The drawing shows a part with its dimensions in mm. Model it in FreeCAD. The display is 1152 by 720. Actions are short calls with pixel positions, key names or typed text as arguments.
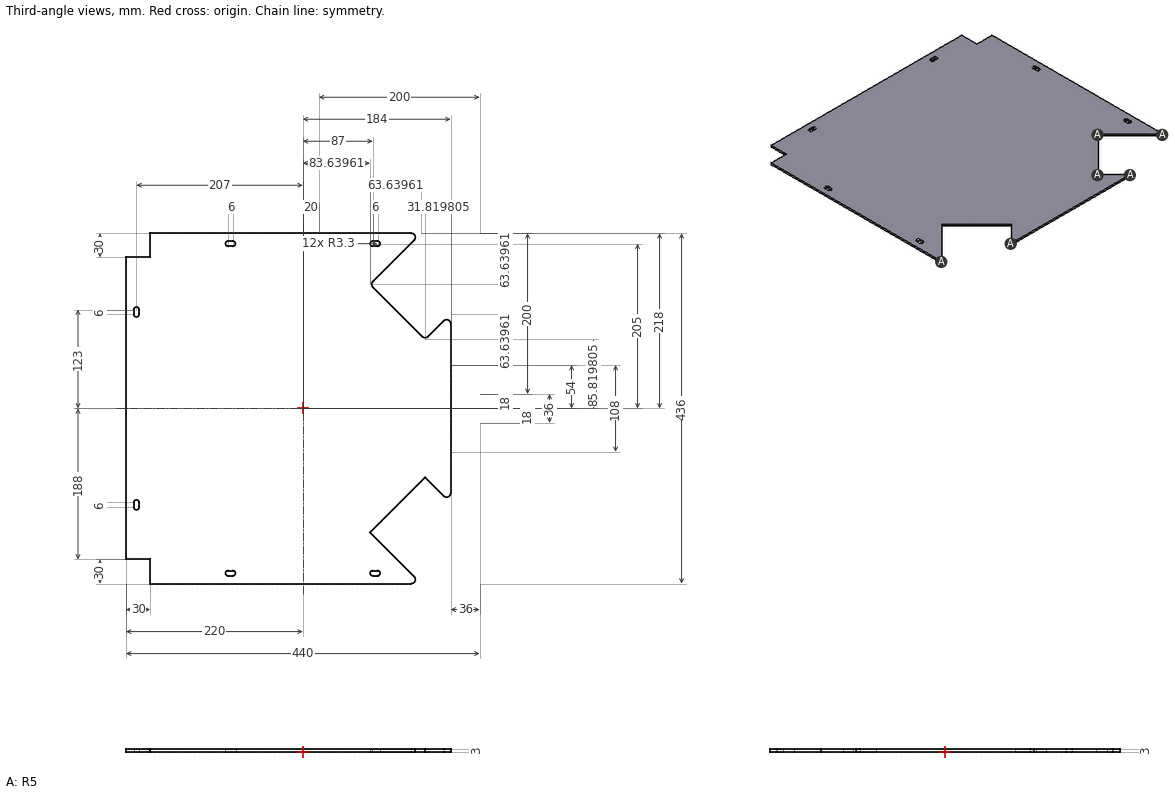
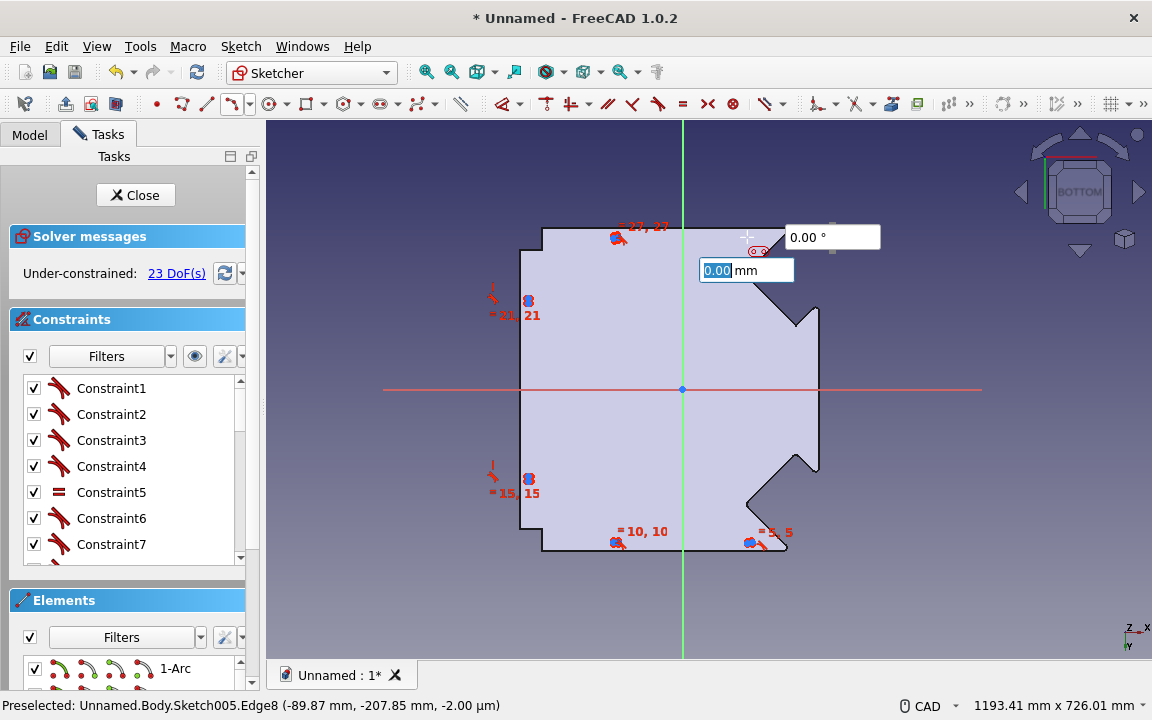
scroll(752, 237, up, 7)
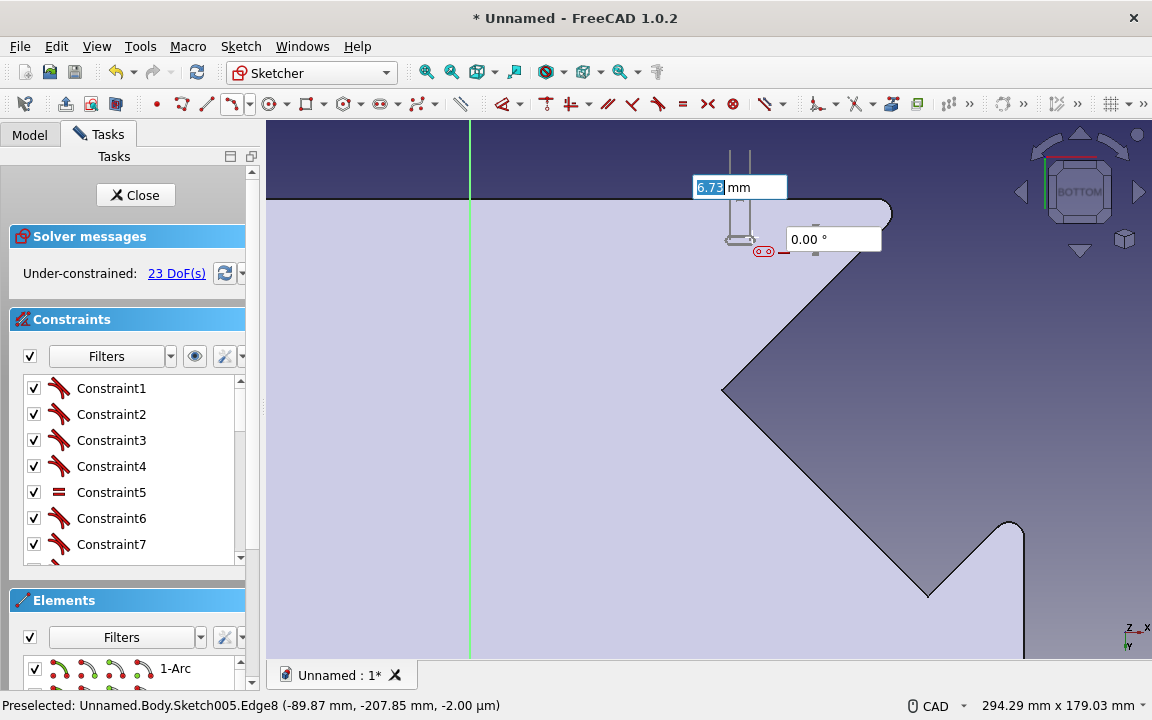
click(750, 236)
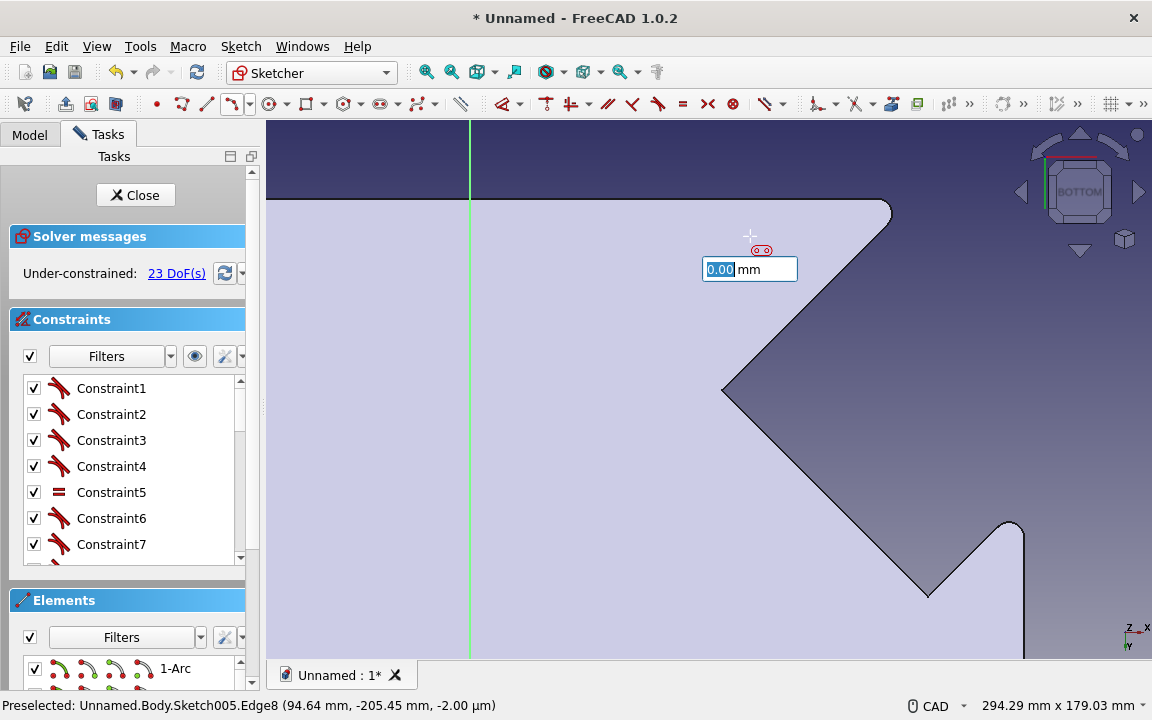
scroll(741, 248, up, 3)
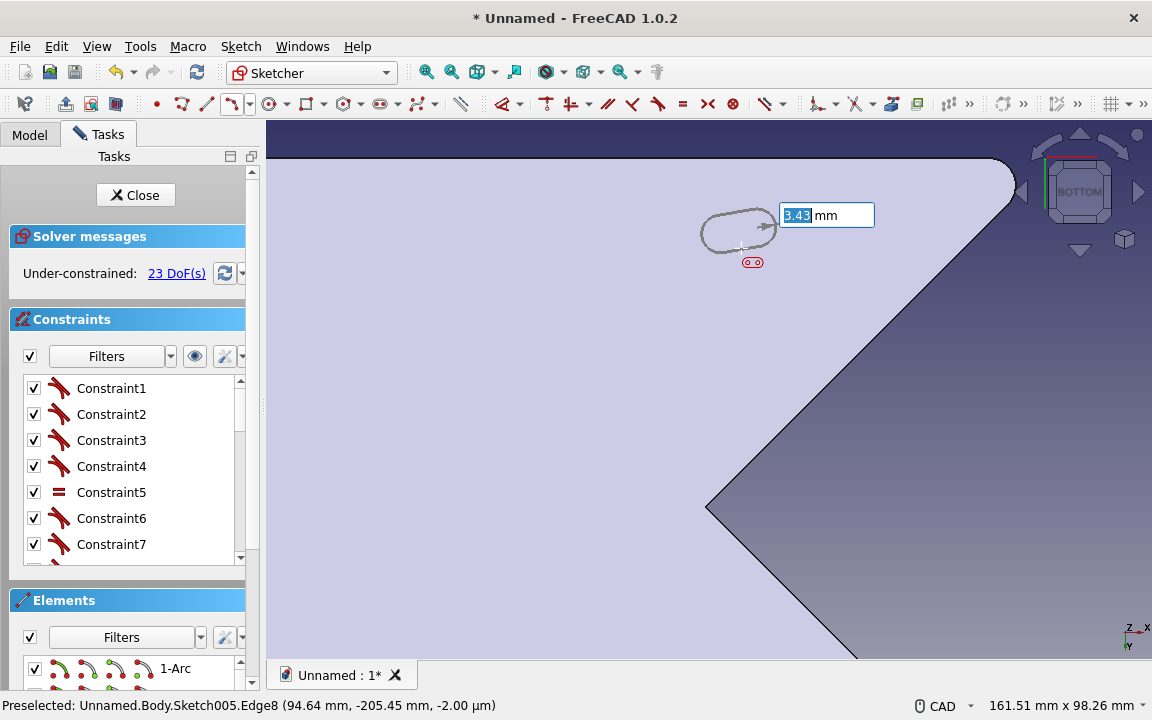
click(740, 247)
key(Escape)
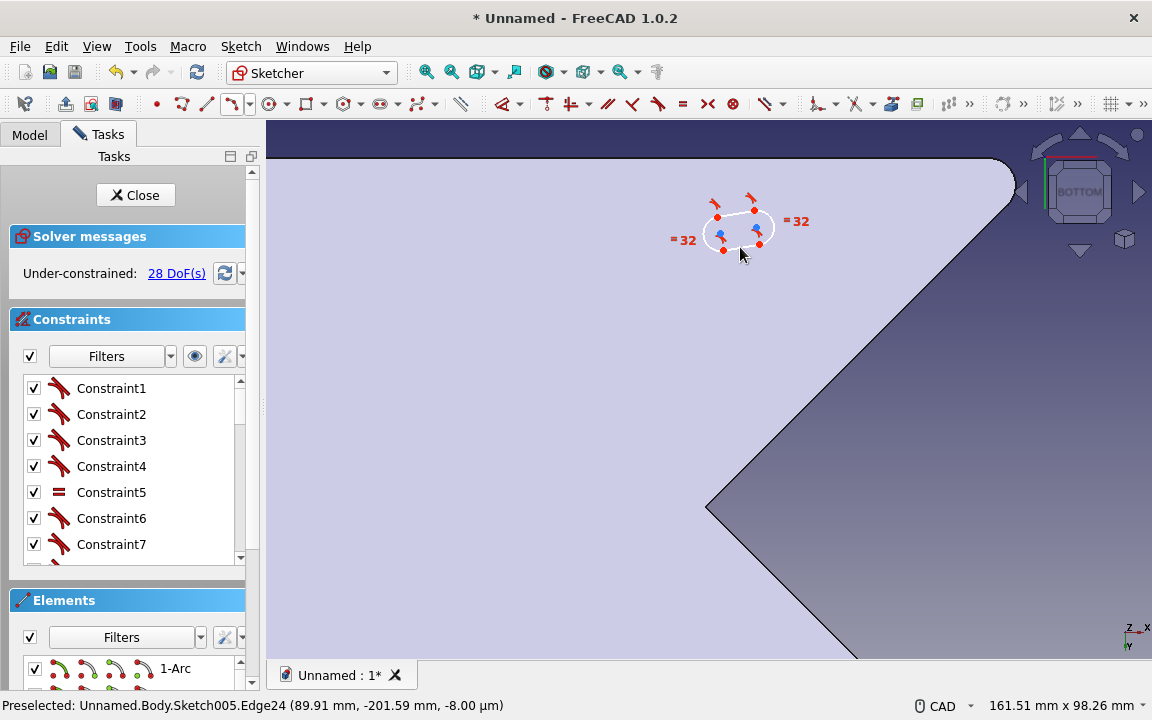
scroll(751, 239, down, 10)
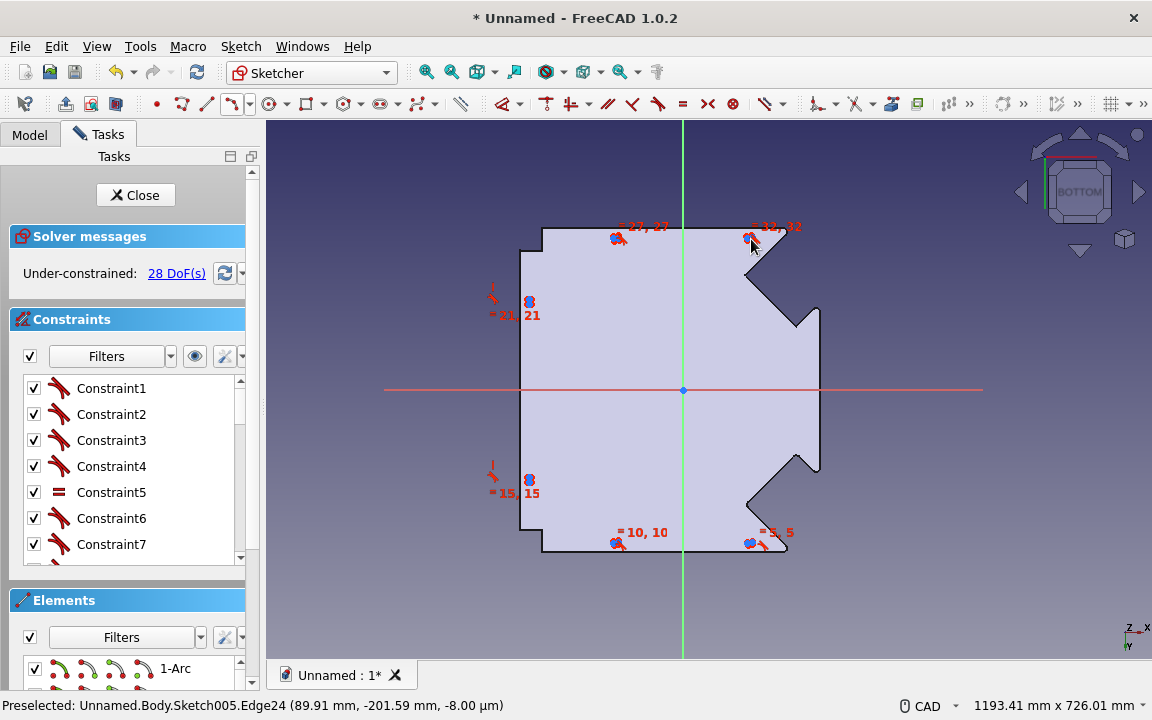
scroll(749, 542, up, 12)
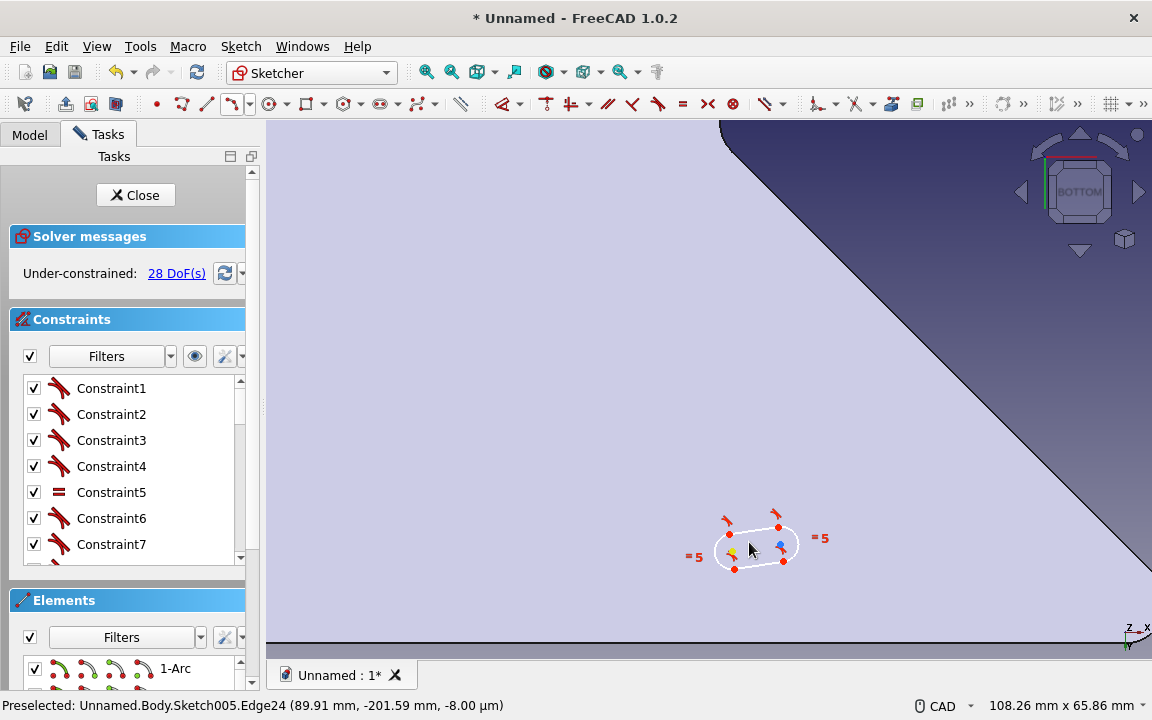
click(744, 532)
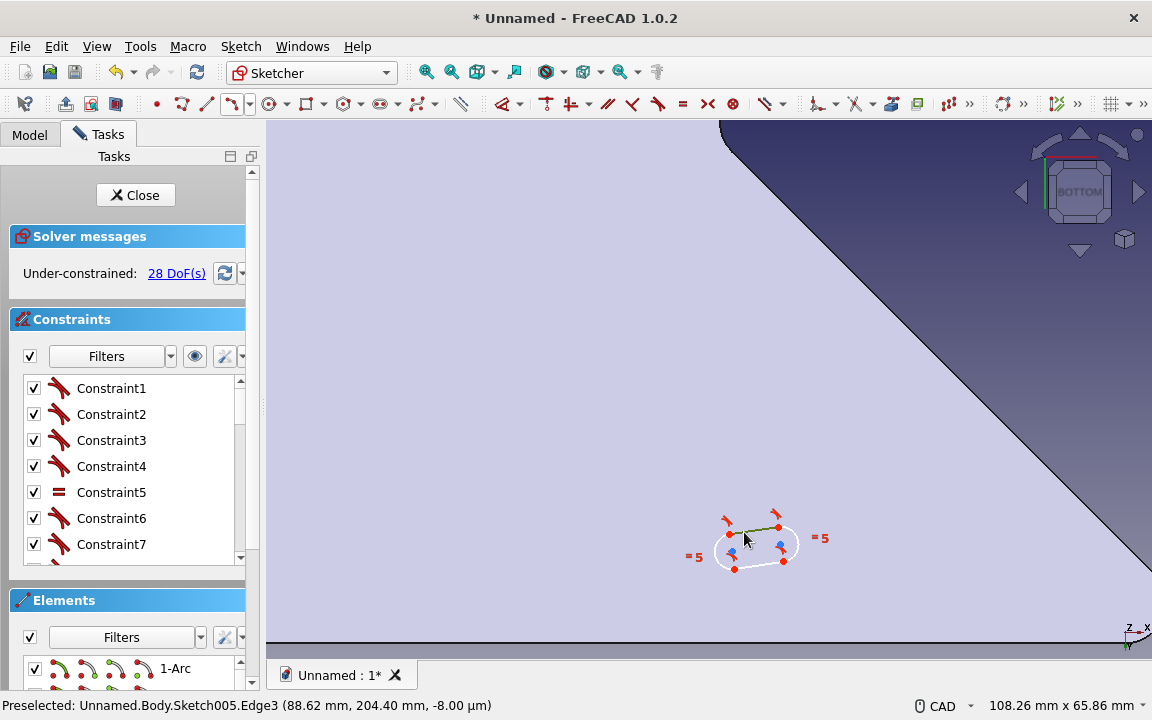
click(588, 104)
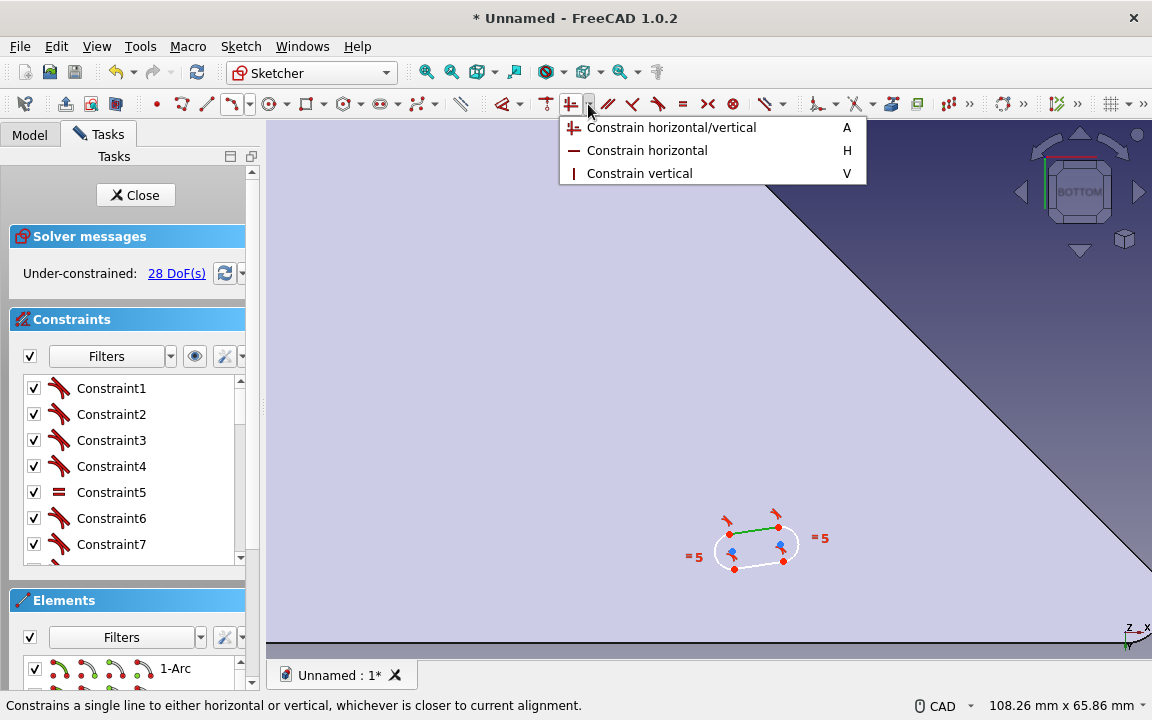
click(713, 150)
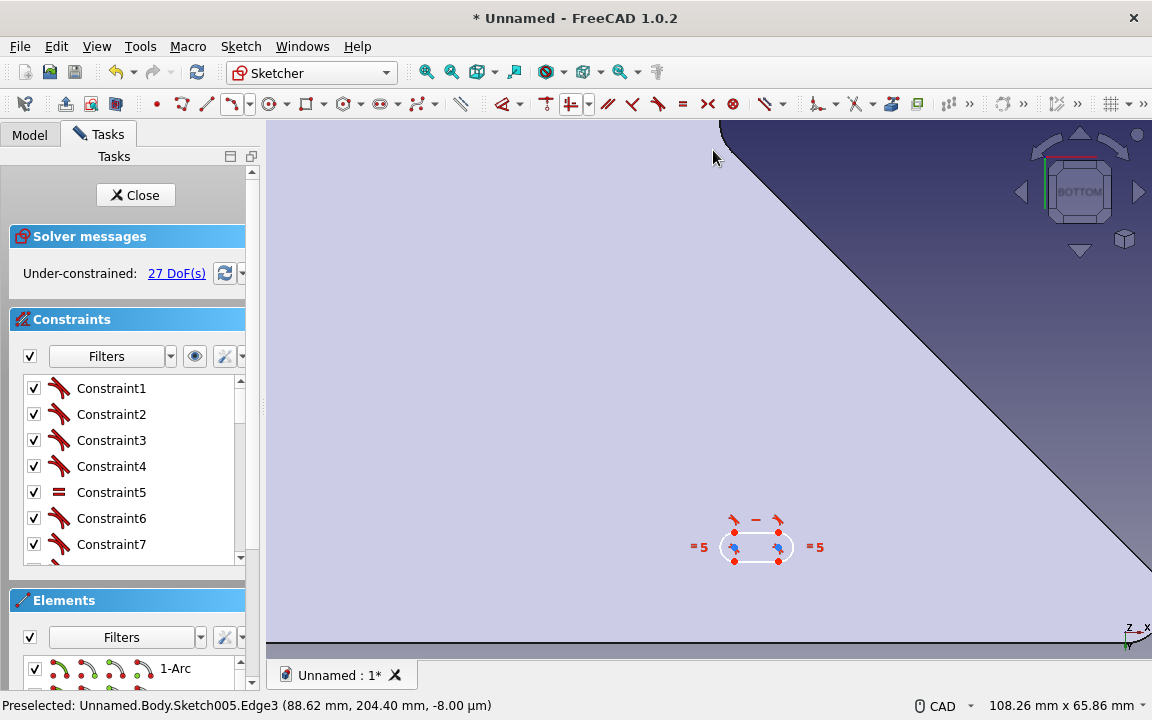
scroll(749, 542, down, 12)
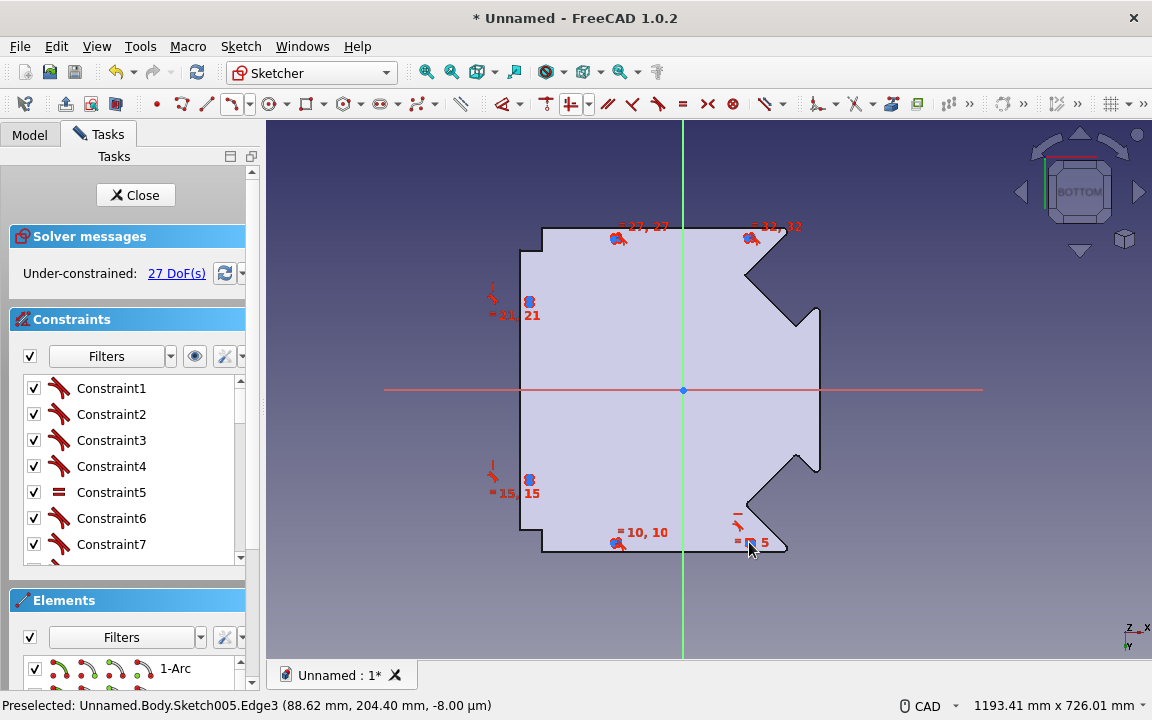
scroll(615, 541, up, 12)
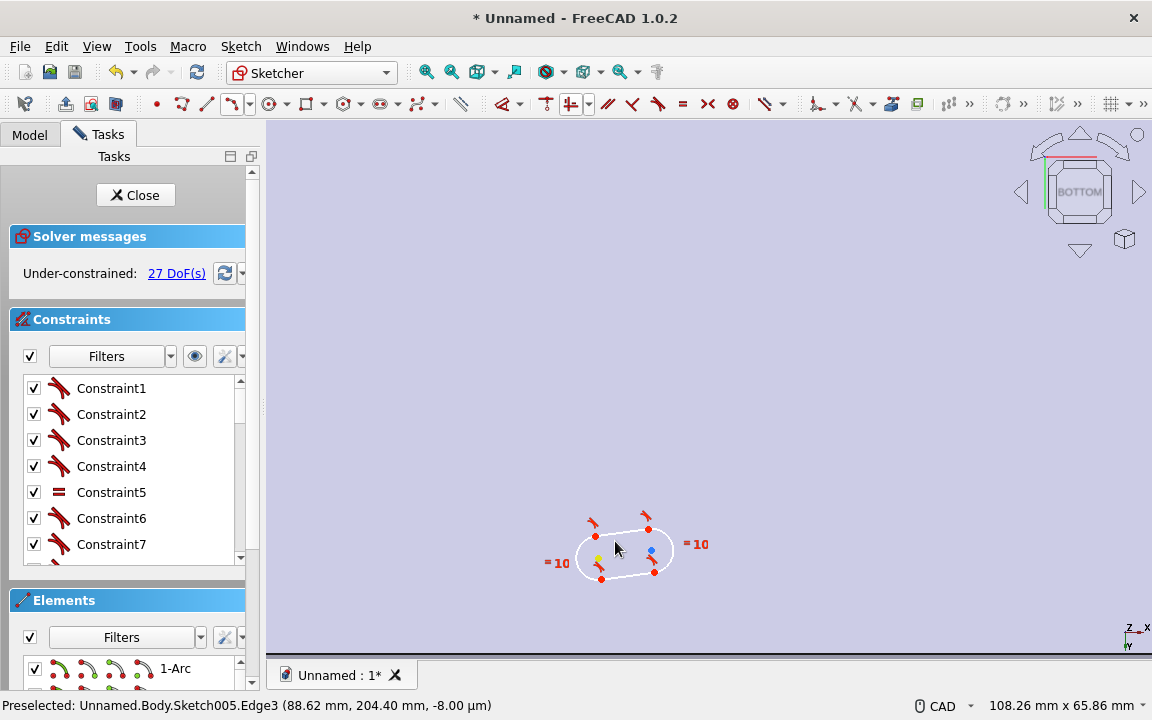
click(611, 534)